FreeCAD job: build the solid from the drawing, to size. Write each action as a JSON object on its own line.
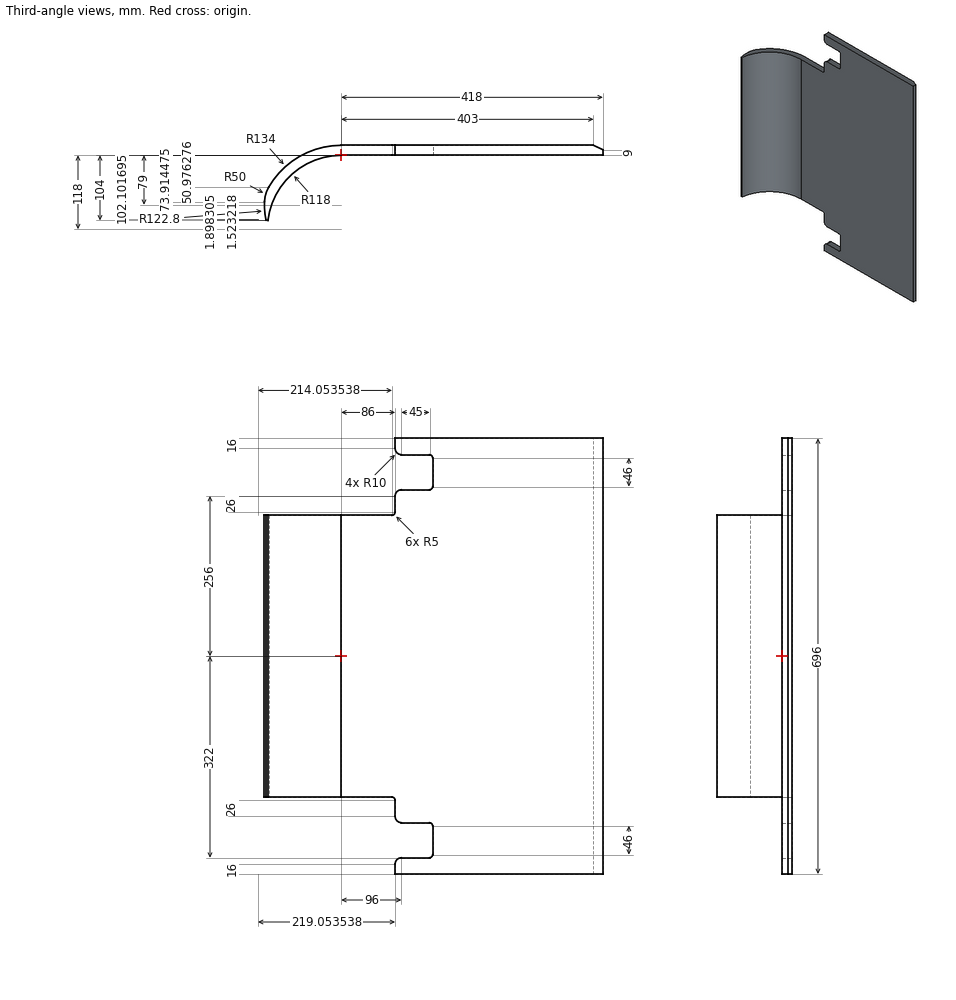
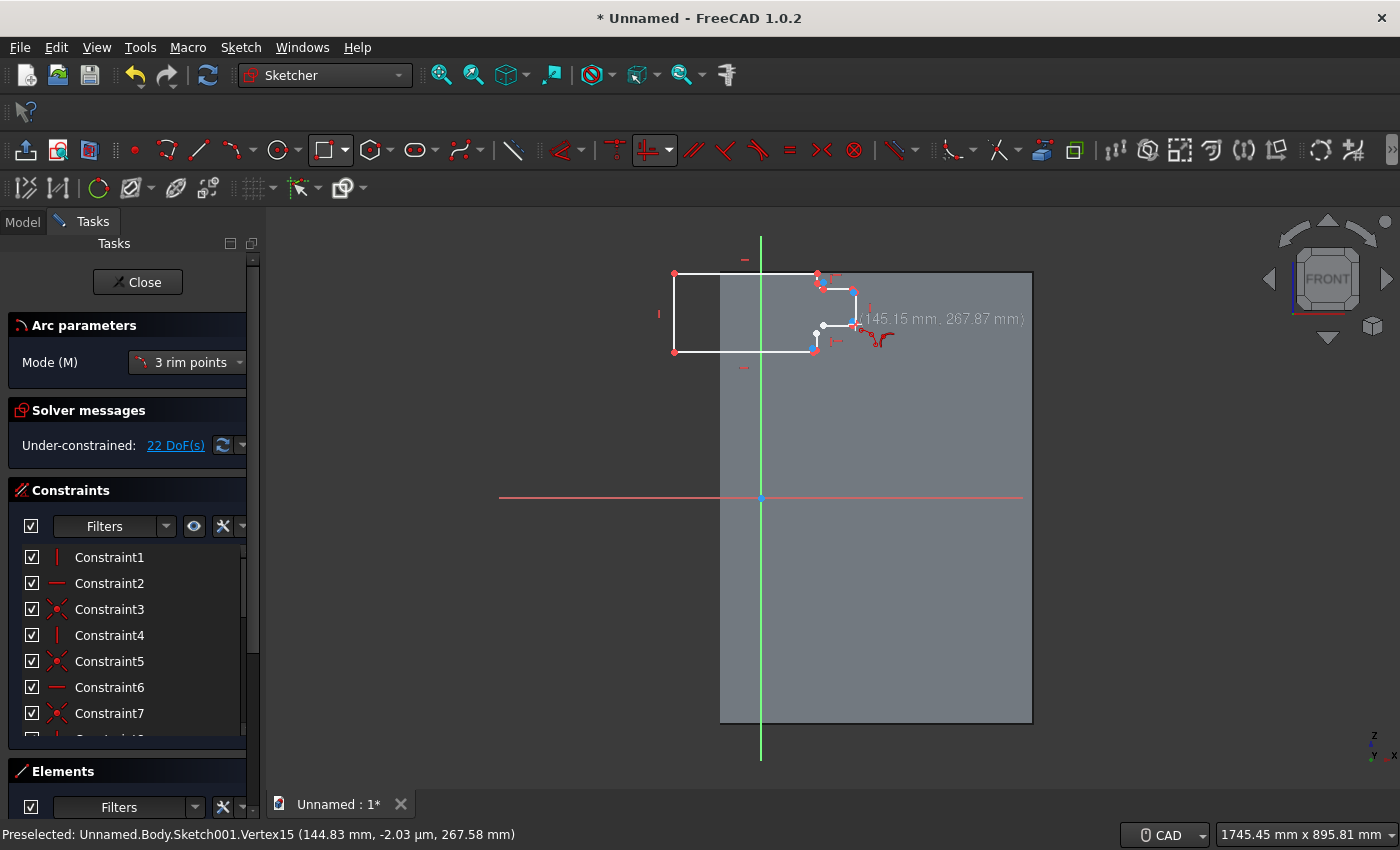
{"action": "scroll", "coordinate": [824, 325], "scroll_direction": "up", "scroll_amount": 3}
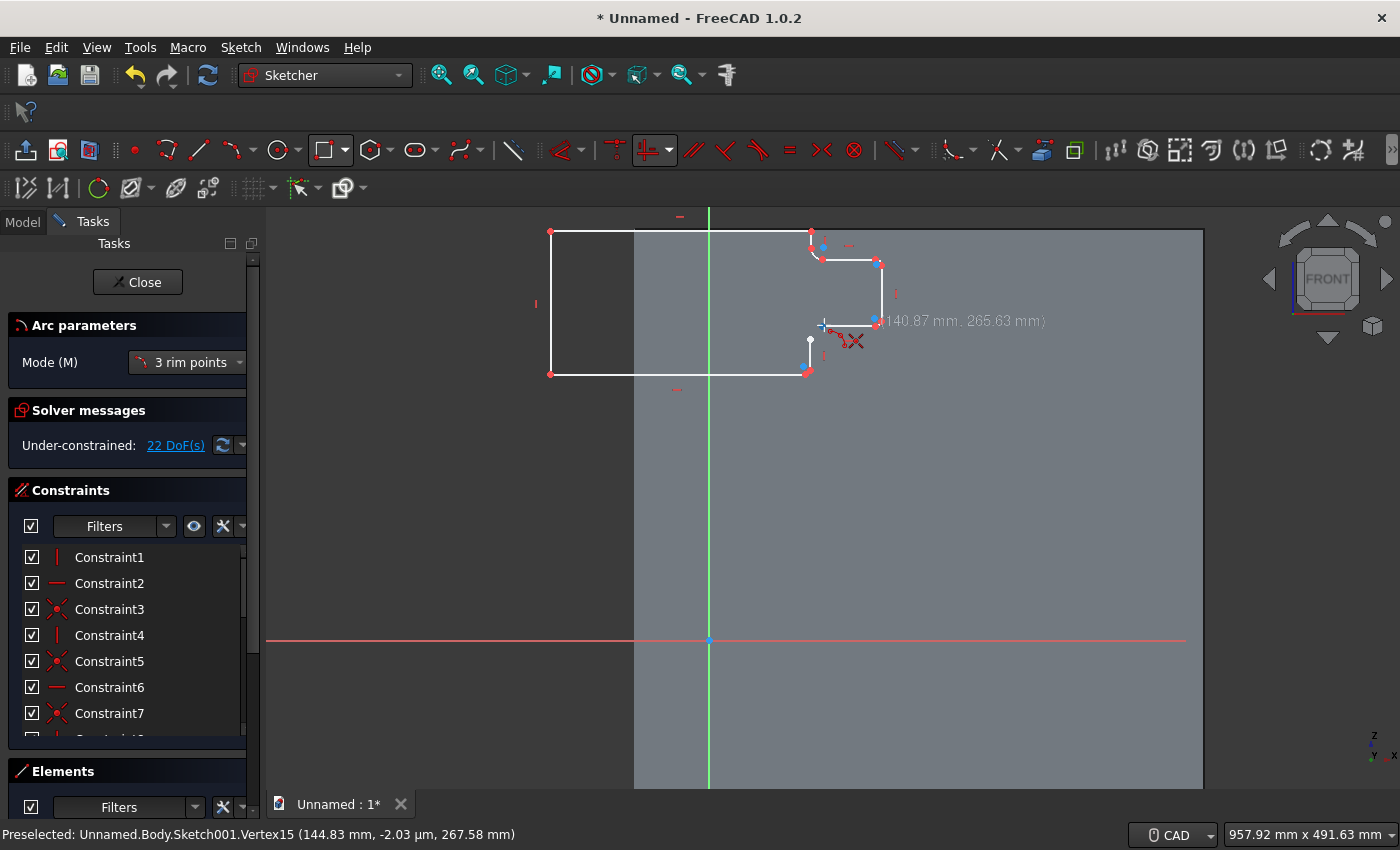
{"action": "left_click", "coordinate": [823, 326]}
{"action": "left_click", "coordinate": [810, 340]}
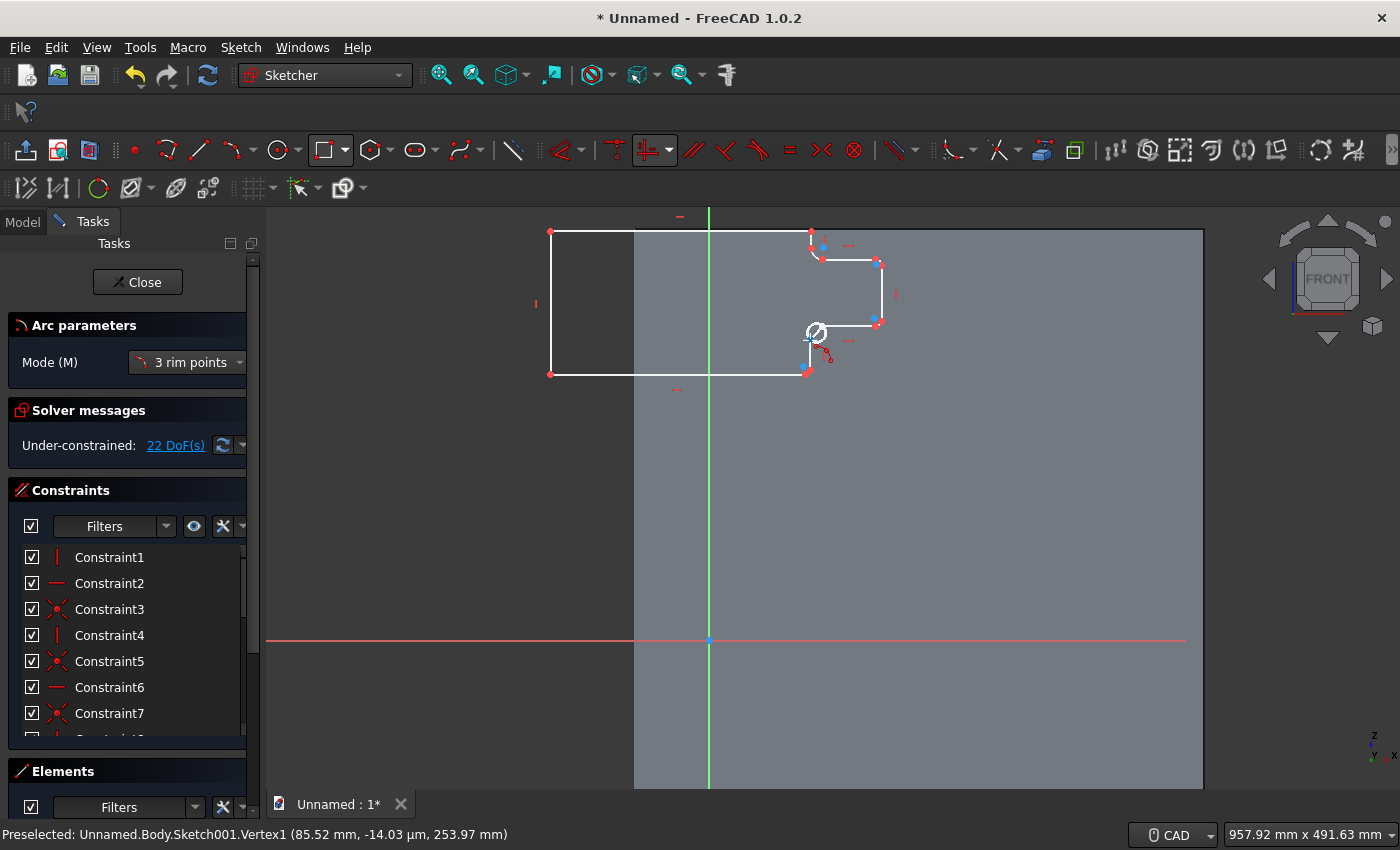
{"action": "scroll", "coordinate": [814, 329], "scroll_direction": "up", "scroll_amount": 8}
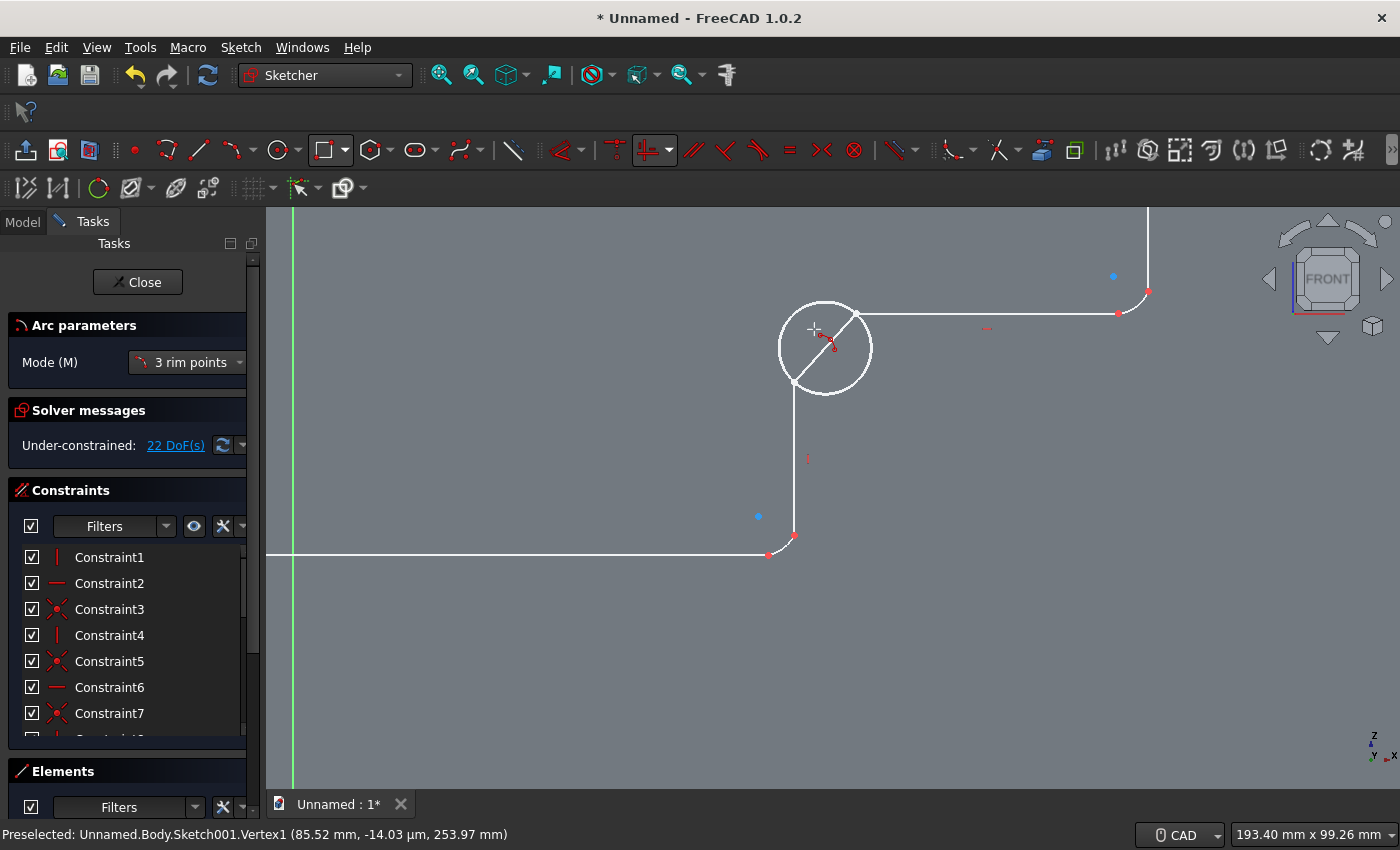
{"action": "left_click", "coordinate": [814, 329]}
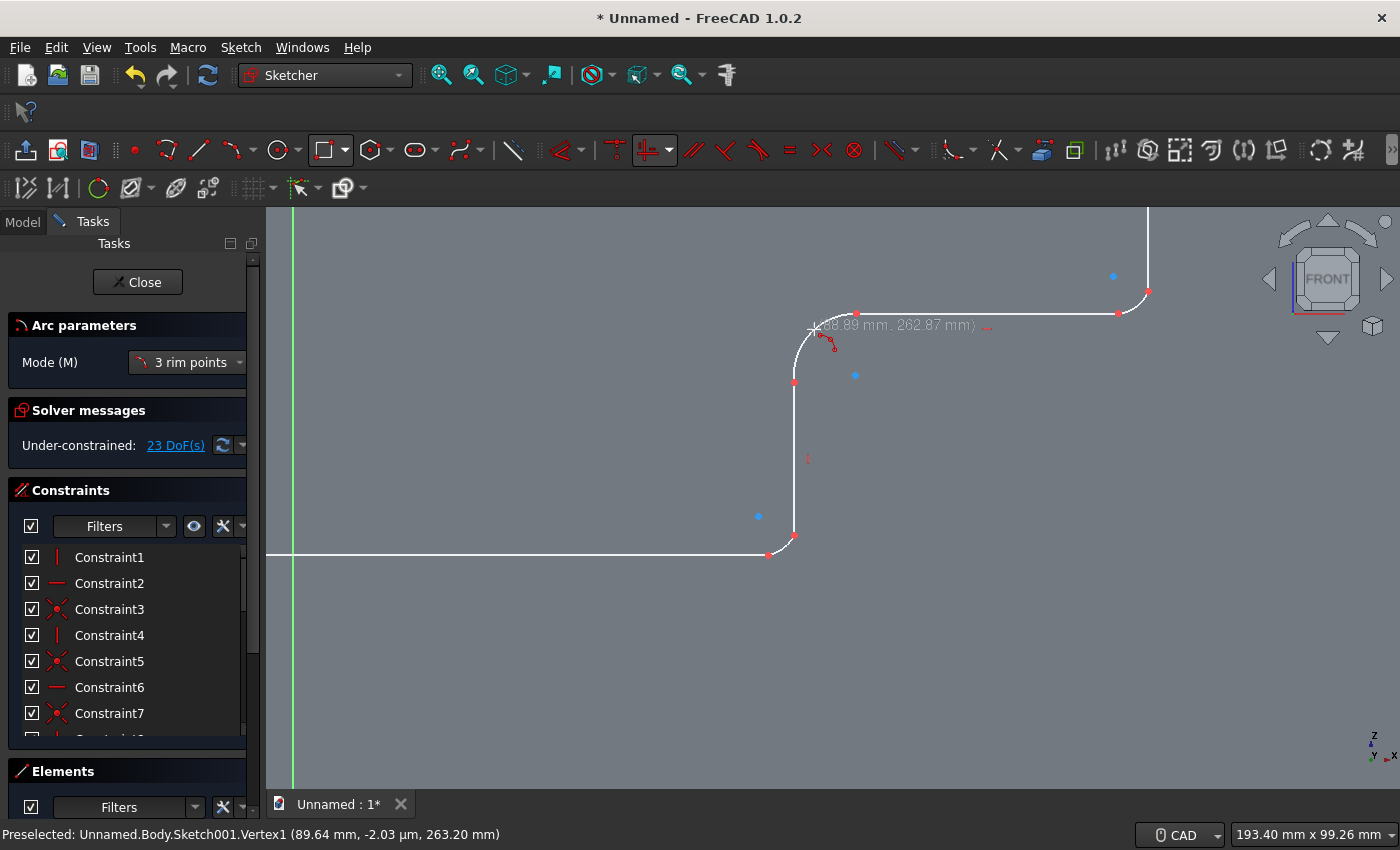
{"action": "left_click", "coordinate": [200, 150]}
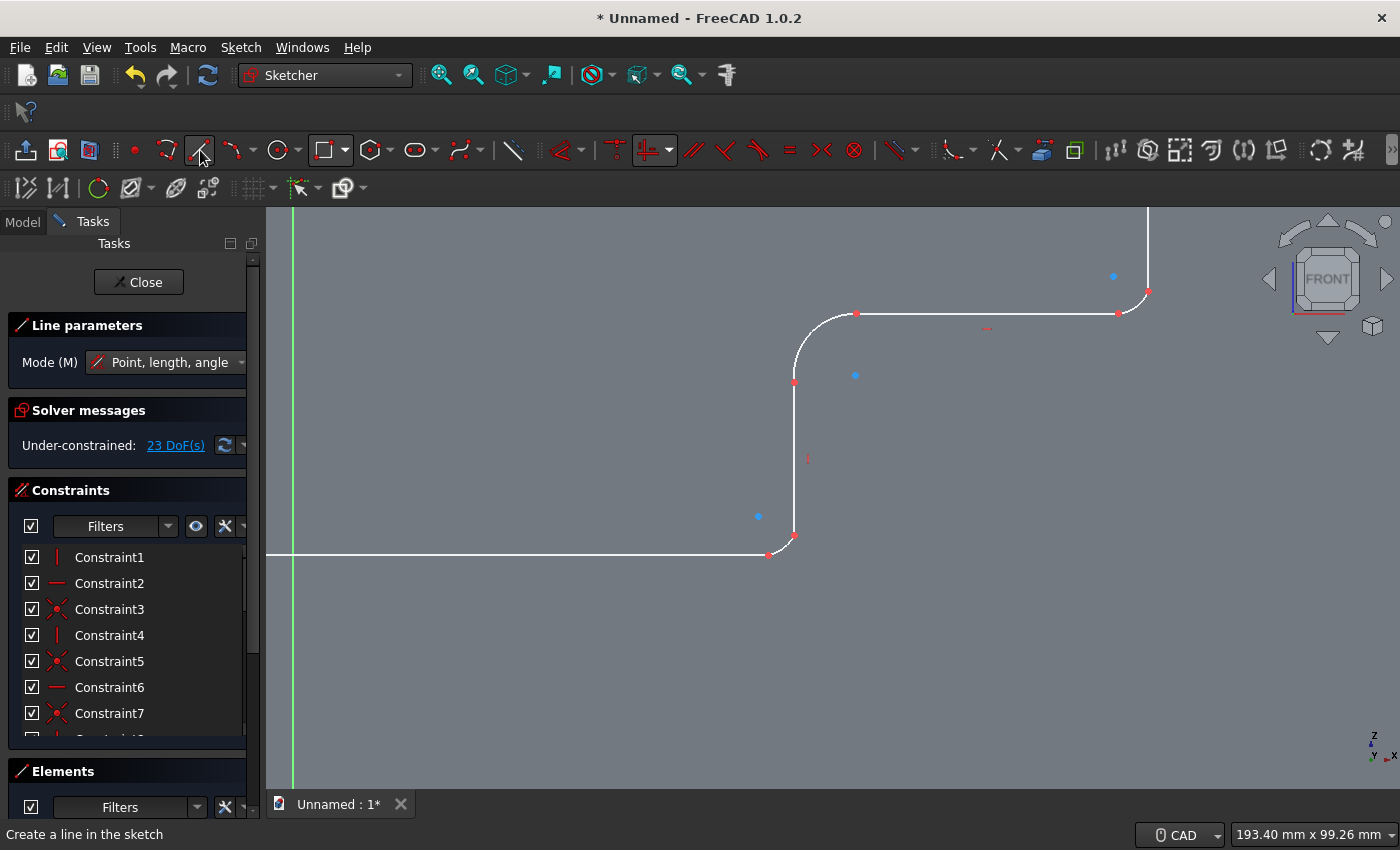
{"action": "scroll", "coordinate": [808, 361], "scroll_direction": "down", "scroll_amount": 12}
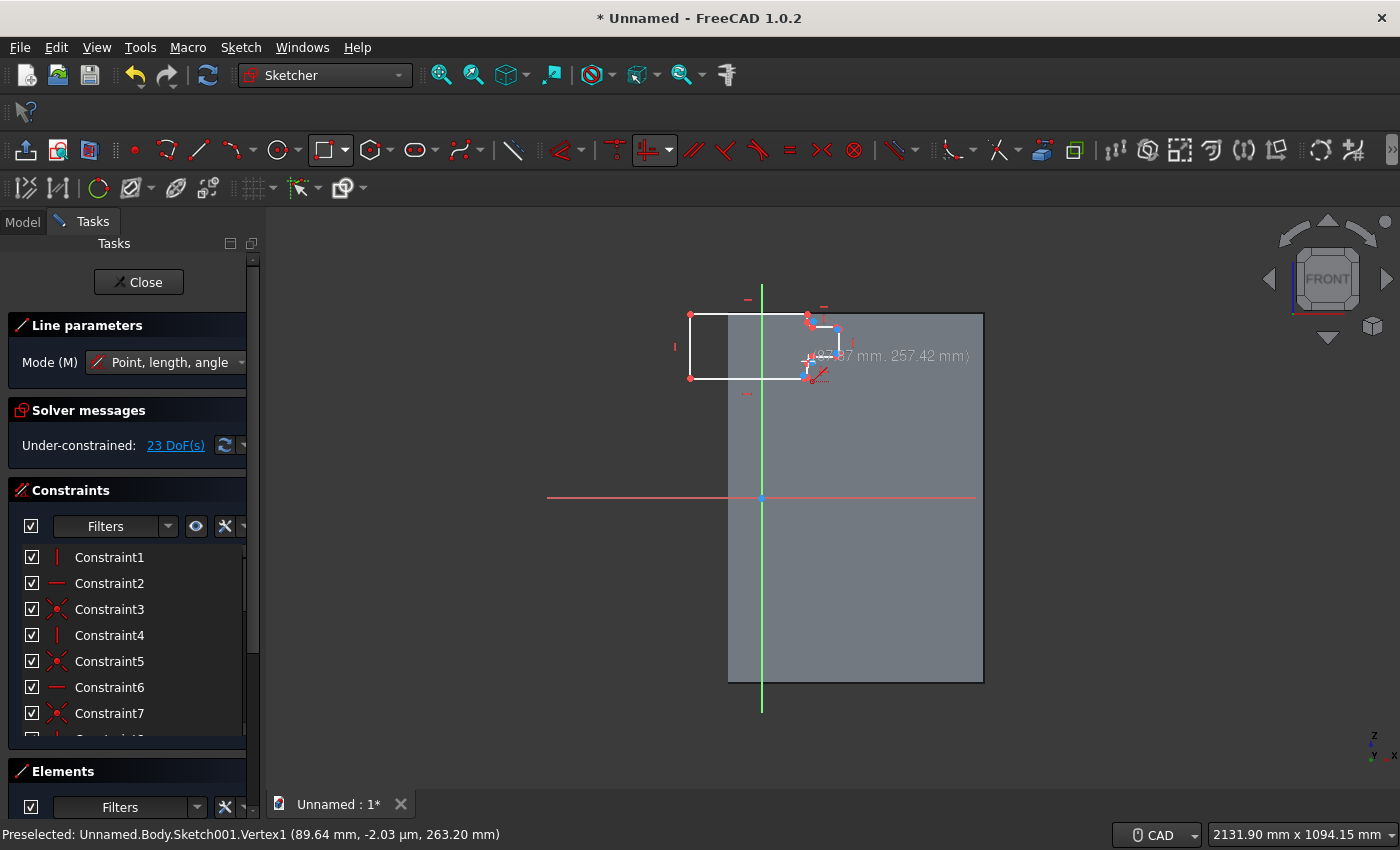
{"action": "left_click", "coordinate": [837, 670]}
{"action": "left_click", "coordinate": [813, 670]}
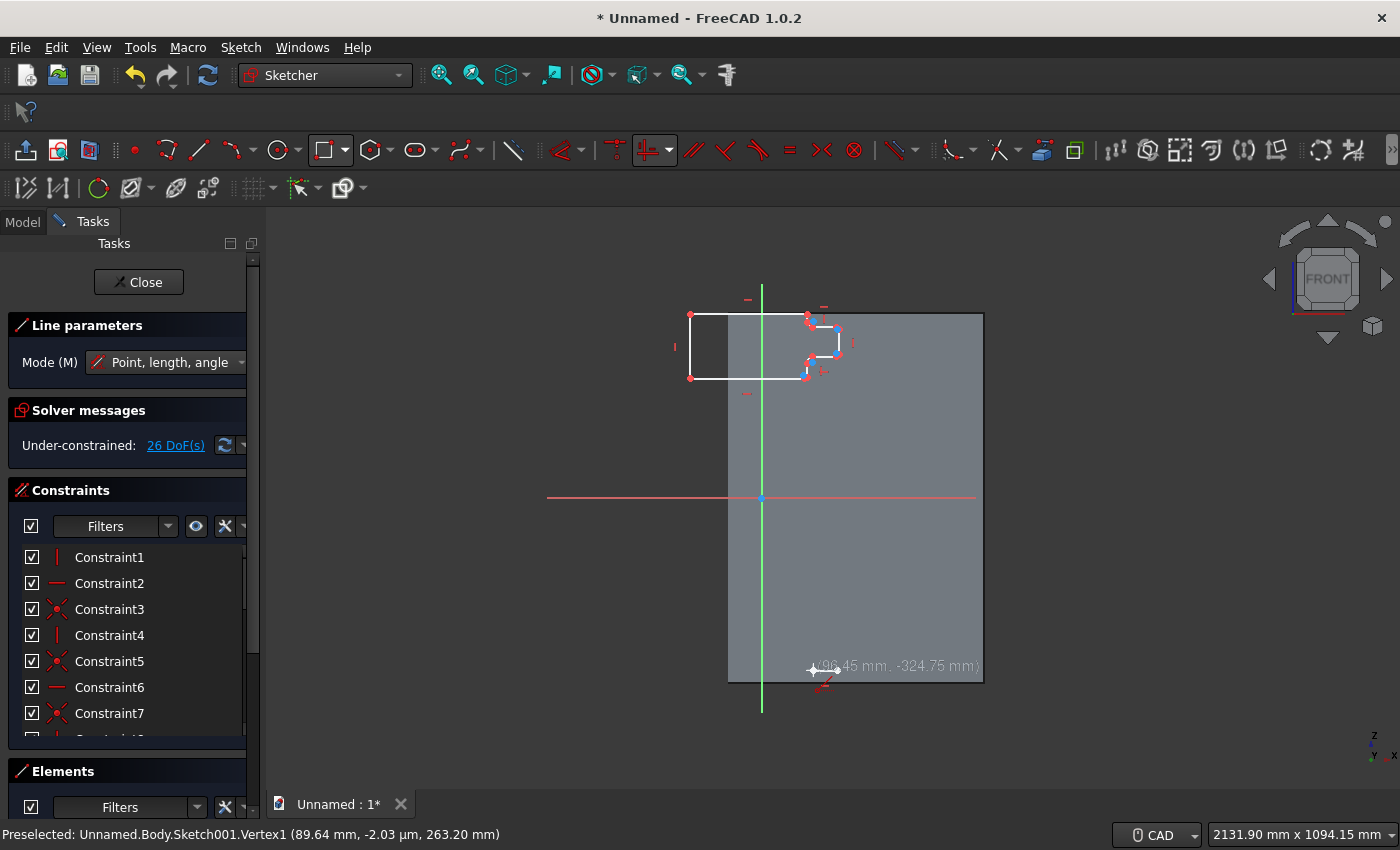
{"action": "left_click", "coordinate": [168, 150]}